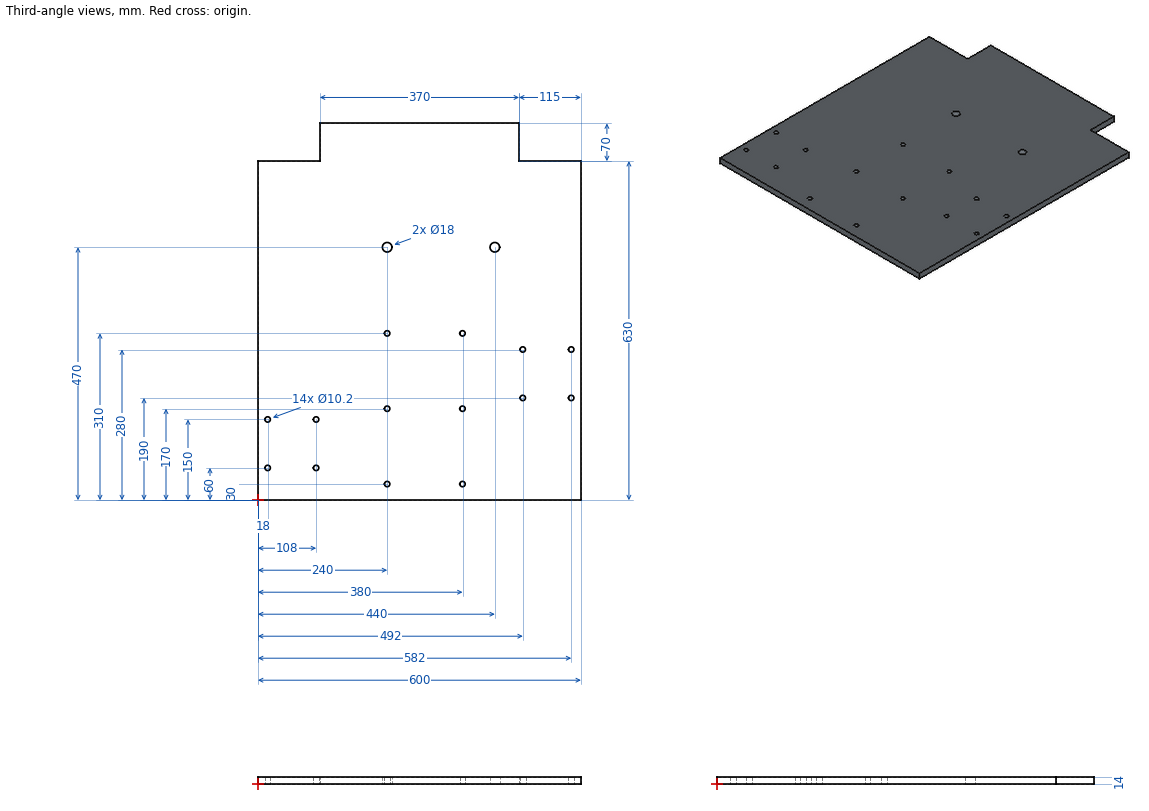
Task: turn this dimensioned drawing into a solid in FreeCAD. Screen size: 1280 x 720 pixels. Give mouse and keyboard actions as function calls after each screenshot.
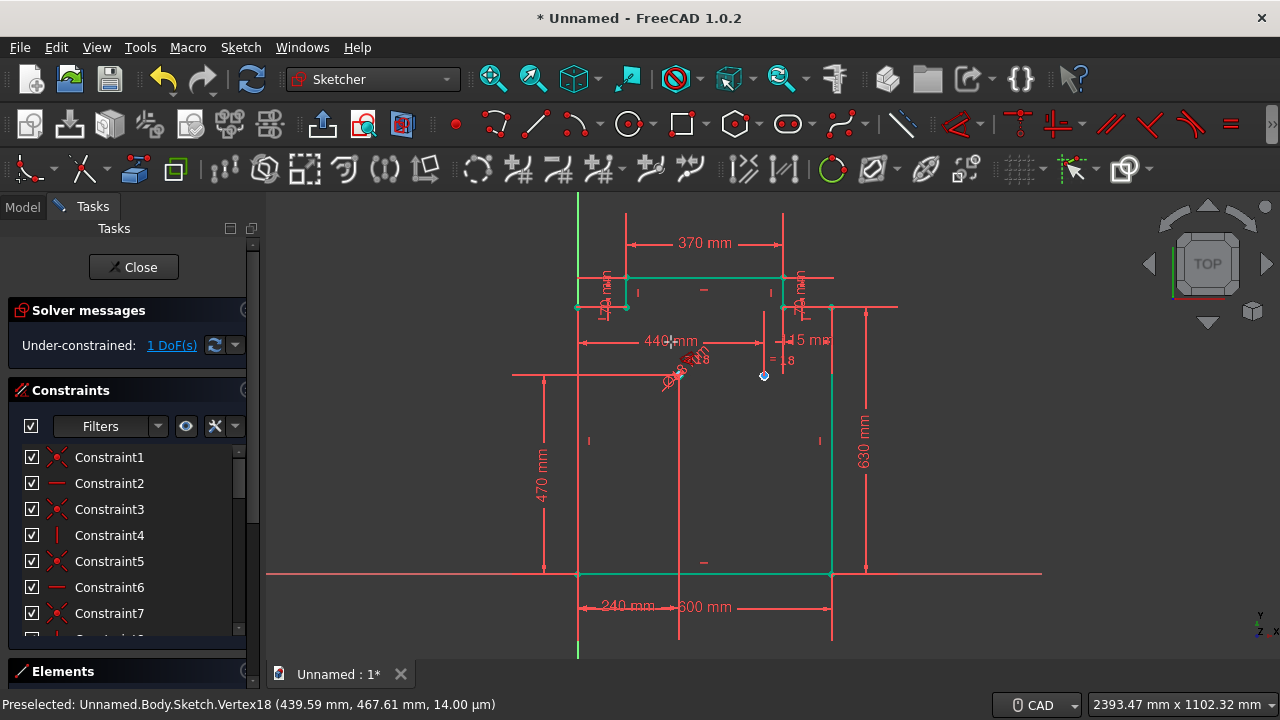
click(764, 376)
click(544, 429)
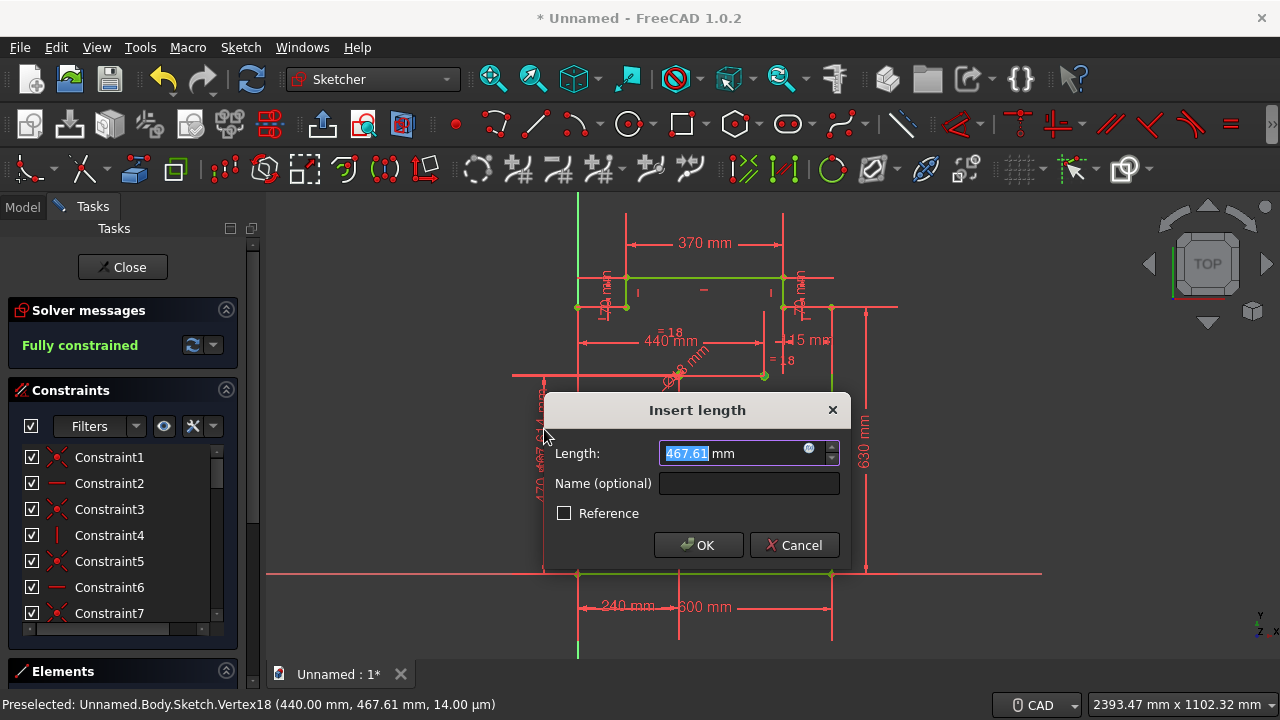
text(470)
key(Return)
key(Escape)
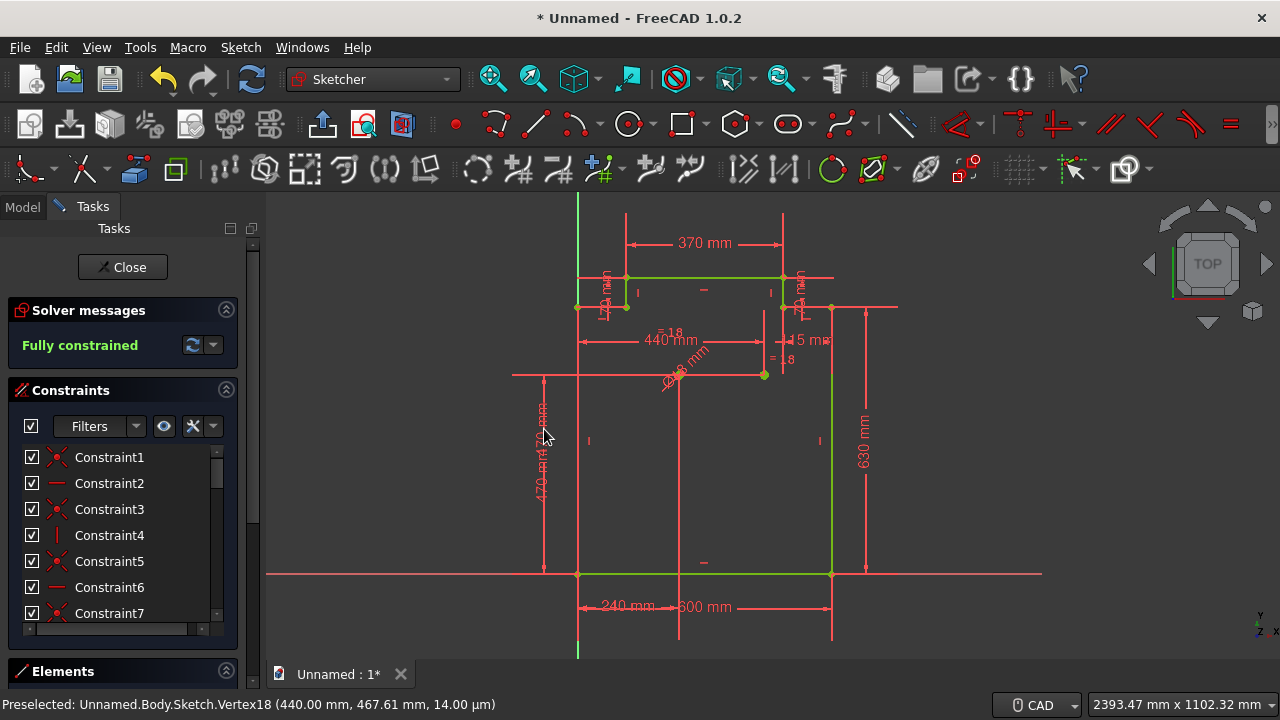
click(123, 267)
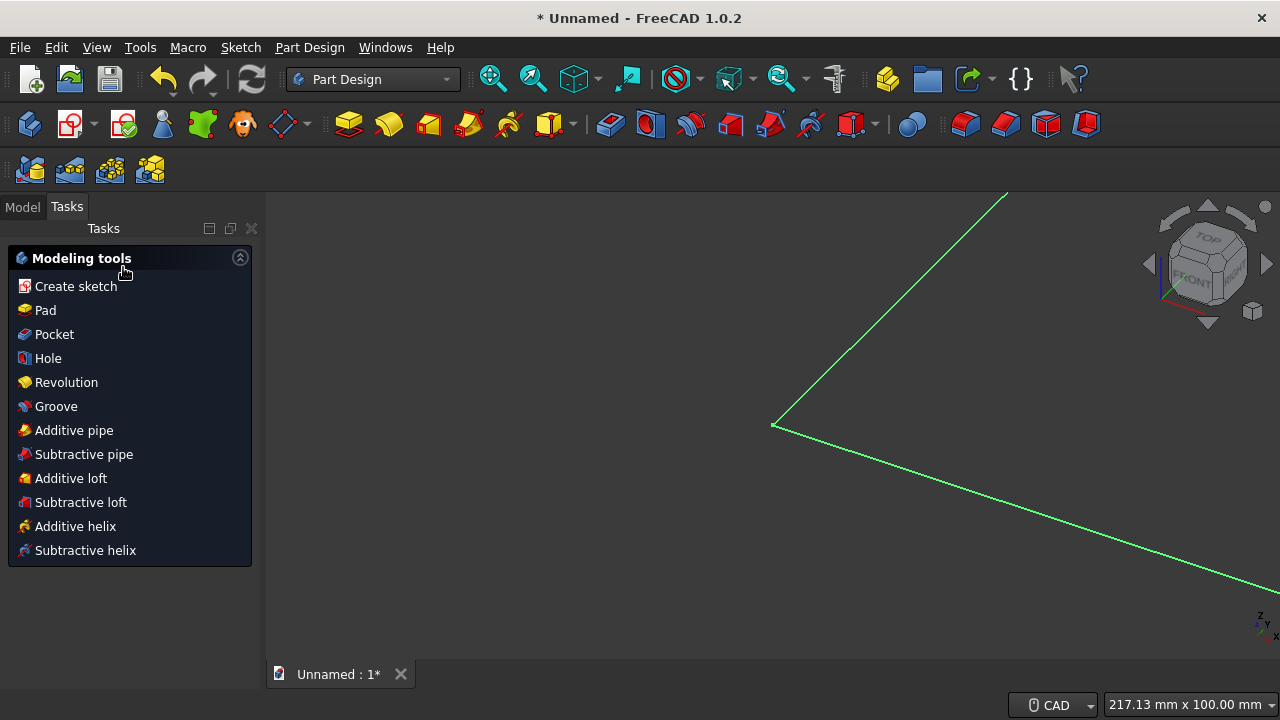
click(350, 124)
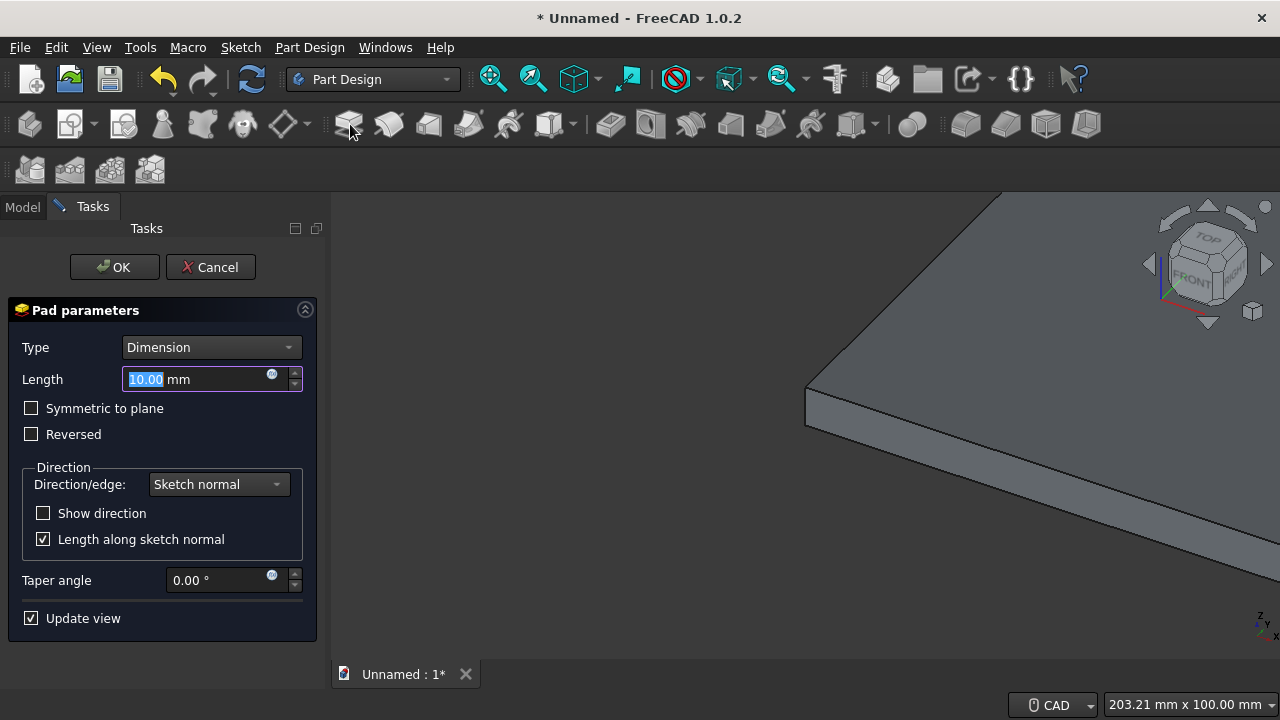
text(14)
key(Tab)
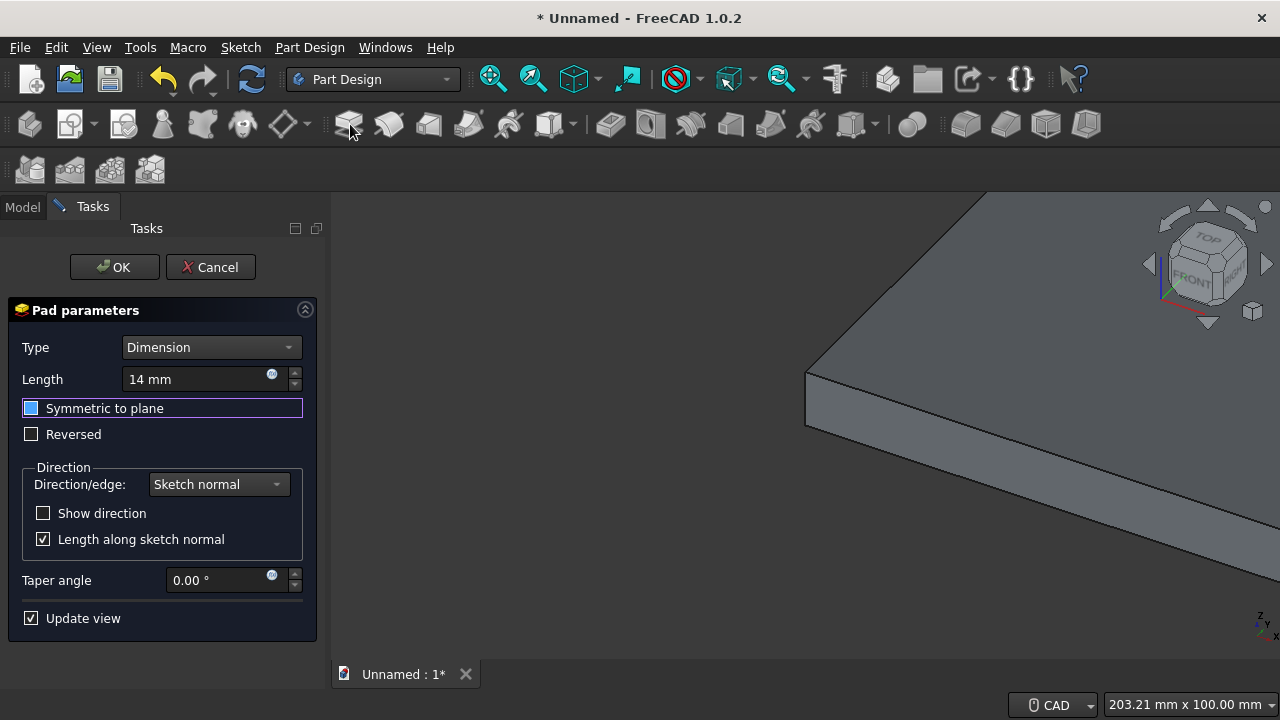
click(115, 267)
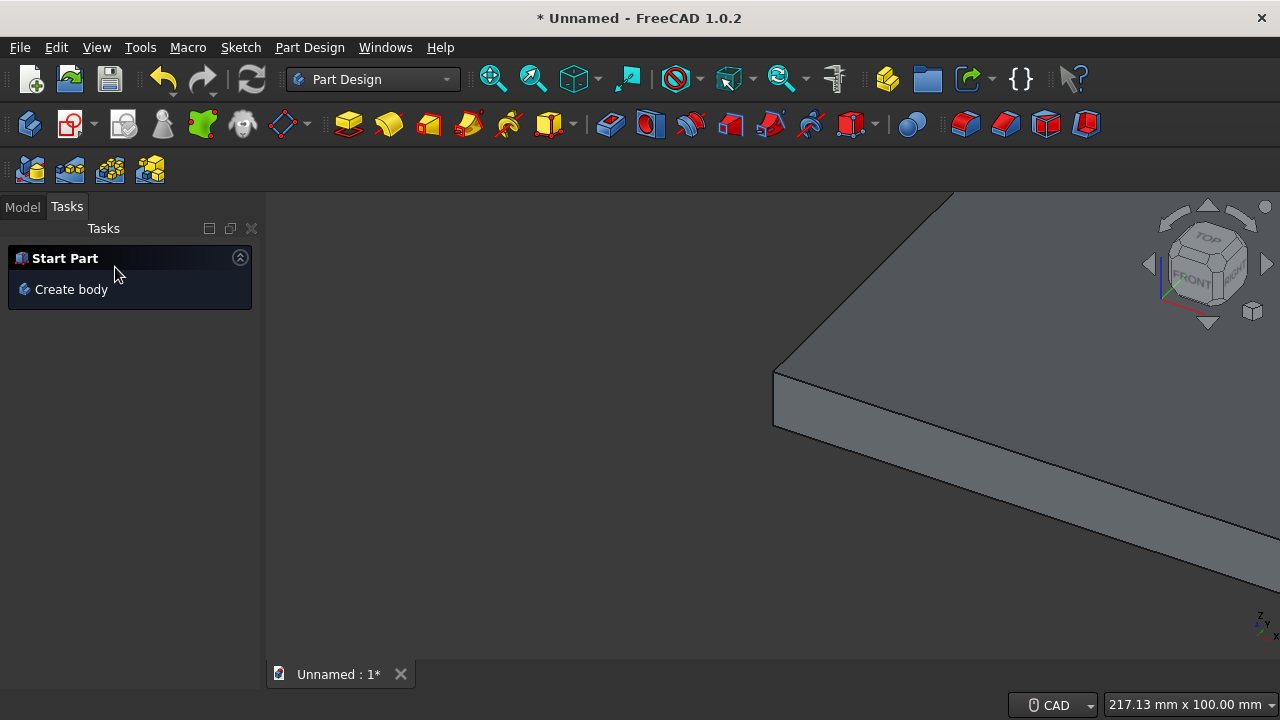
click(494, 80)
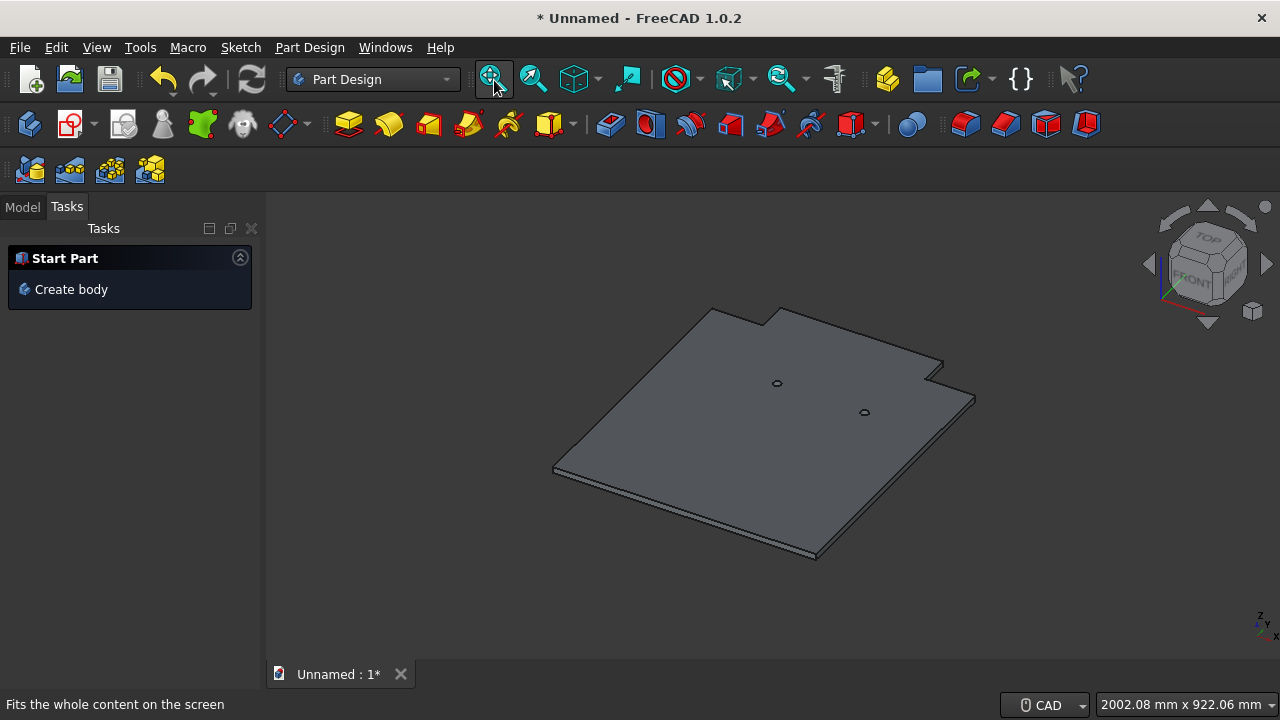
click(748, 447)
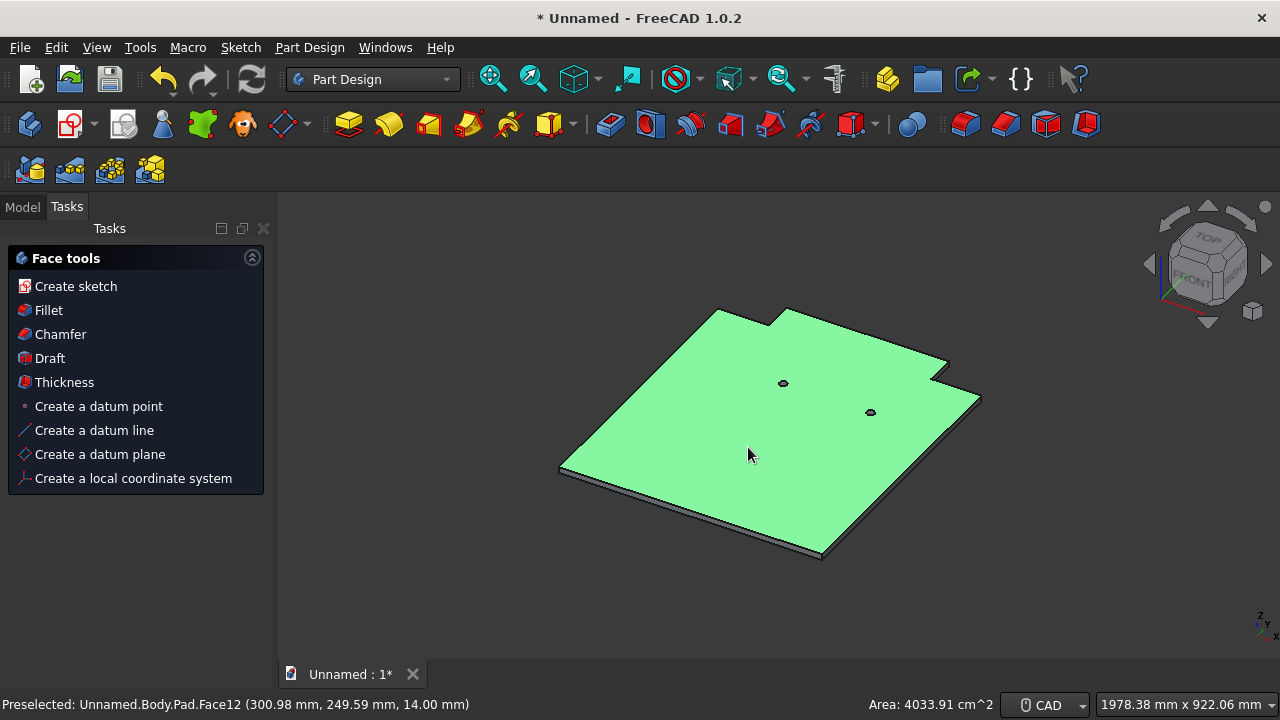
click(70, 124)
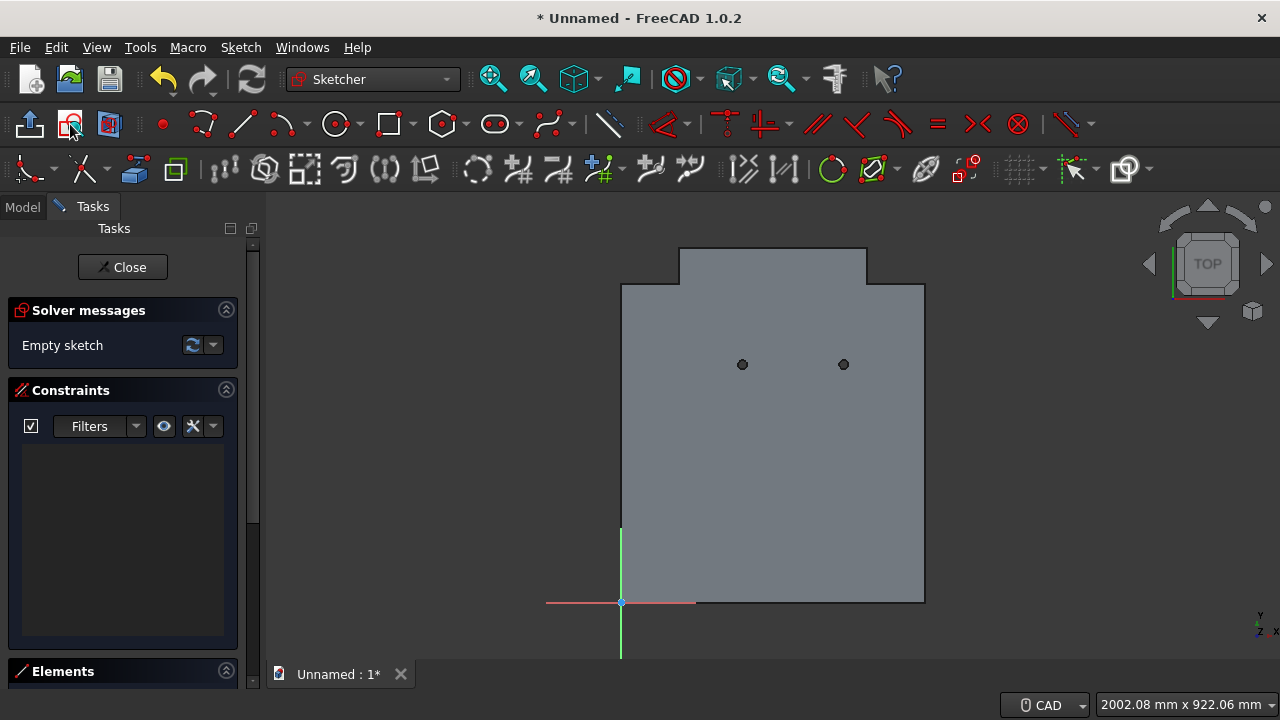
scroll(849, 631, up, 3)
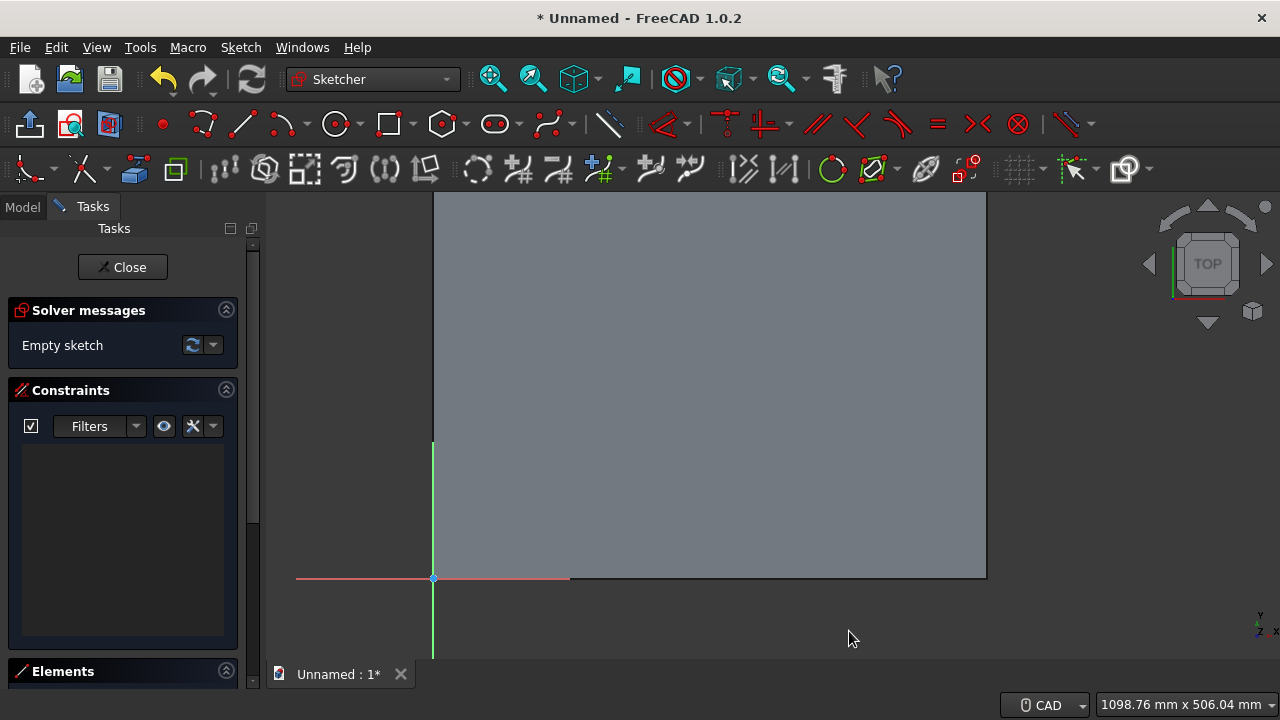
key(g)
key(c)